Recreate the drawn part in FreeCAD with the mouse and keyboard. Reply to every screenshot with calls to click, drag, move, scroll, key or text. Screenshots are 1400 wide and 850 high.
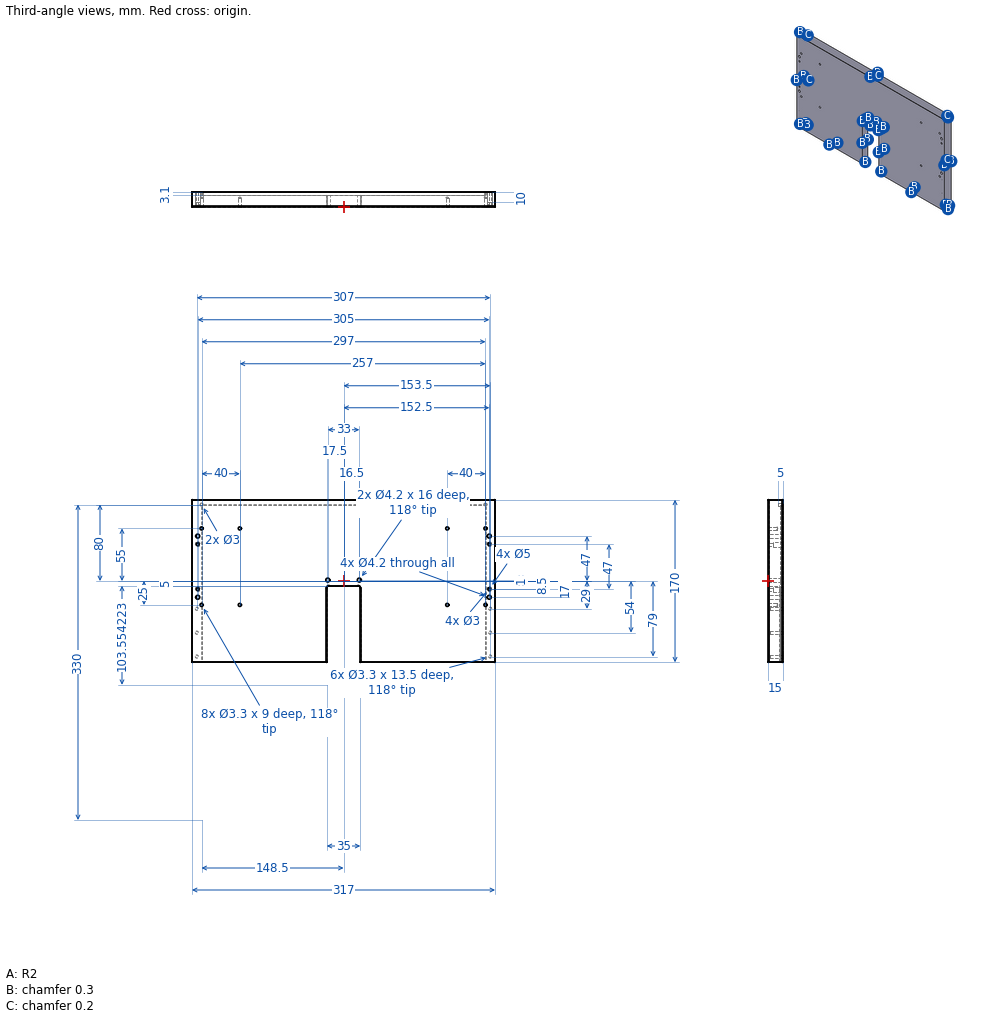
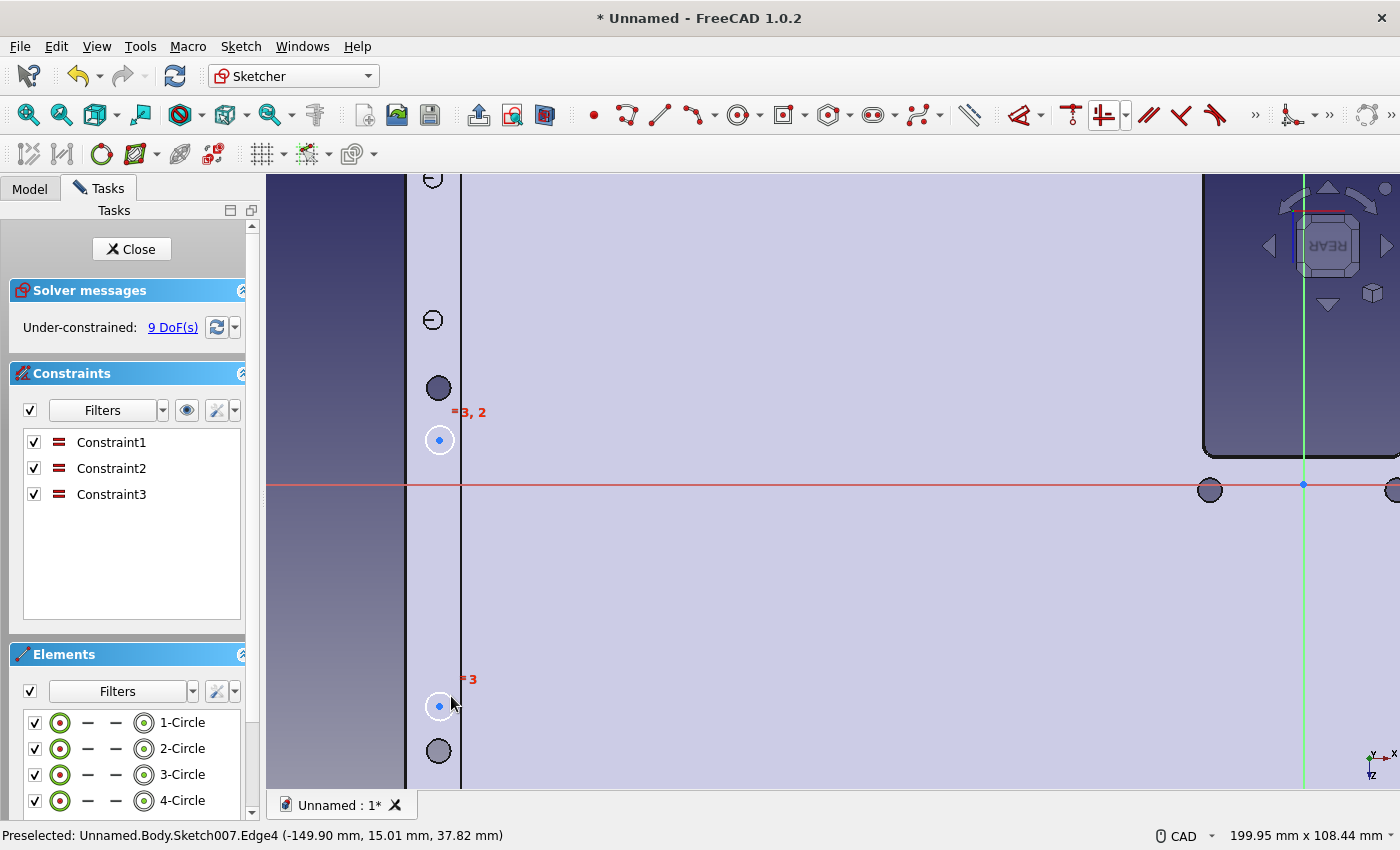
scroll(451, 430, down, 5)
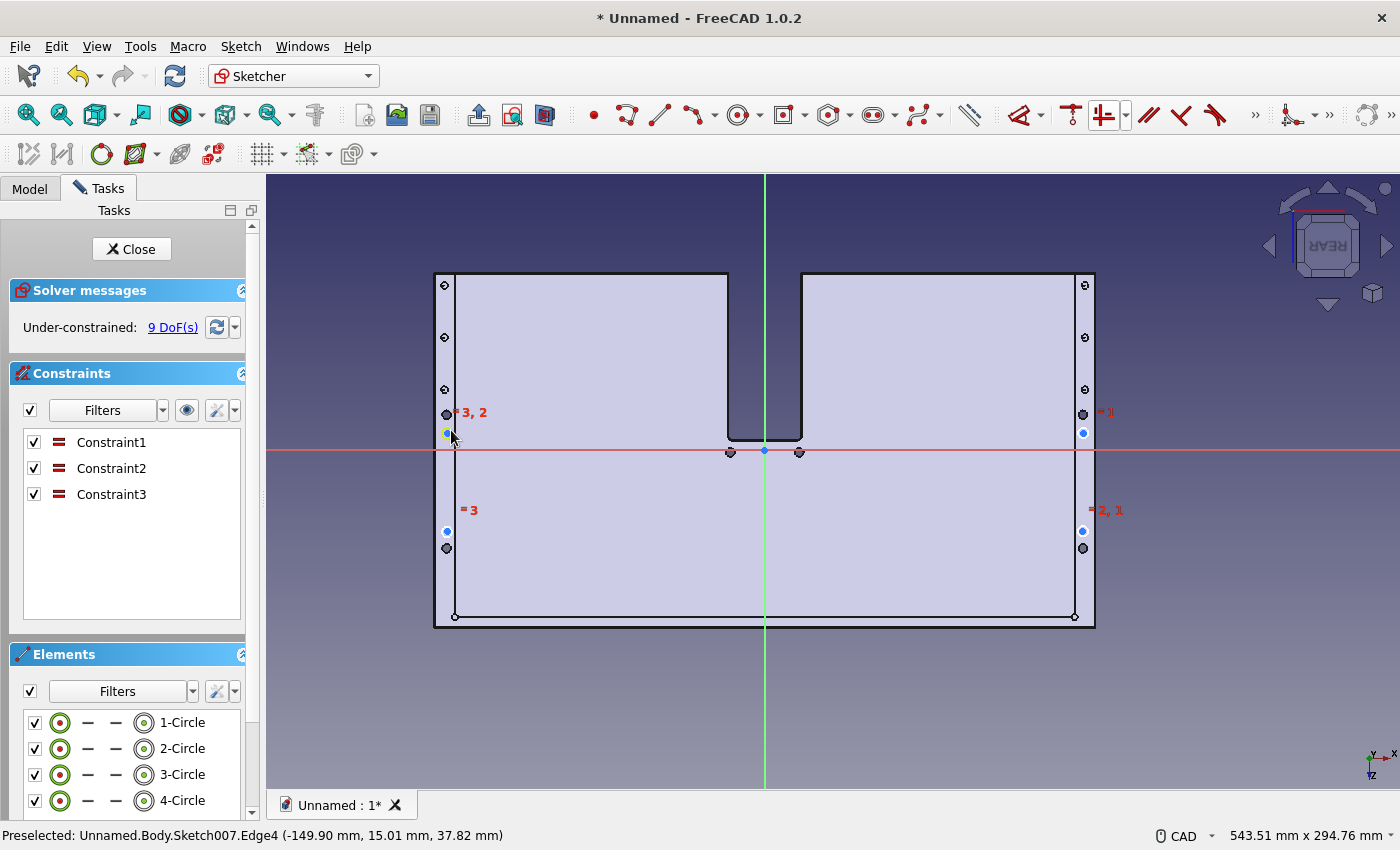
click(1083, 433)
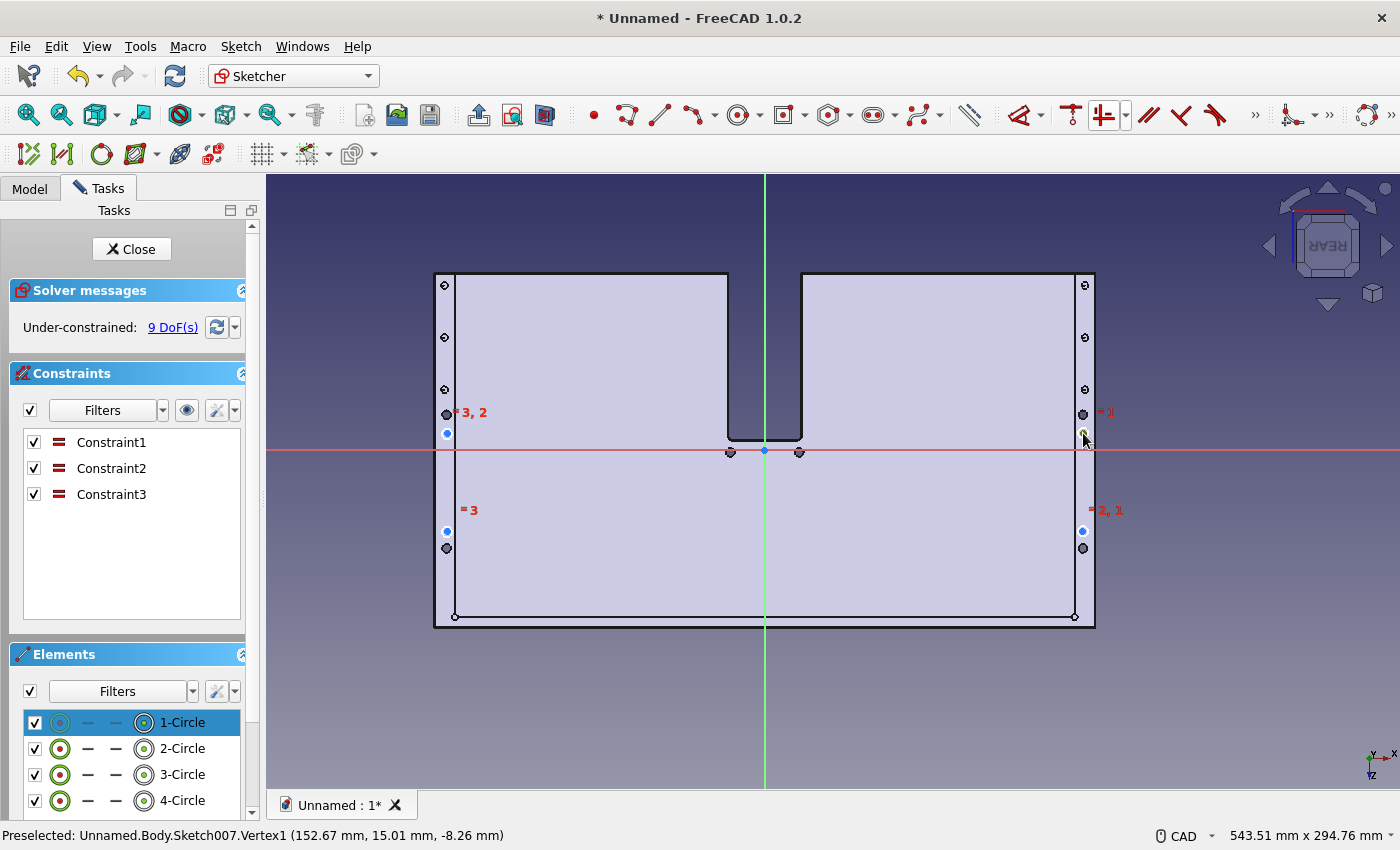
click(1083, 531)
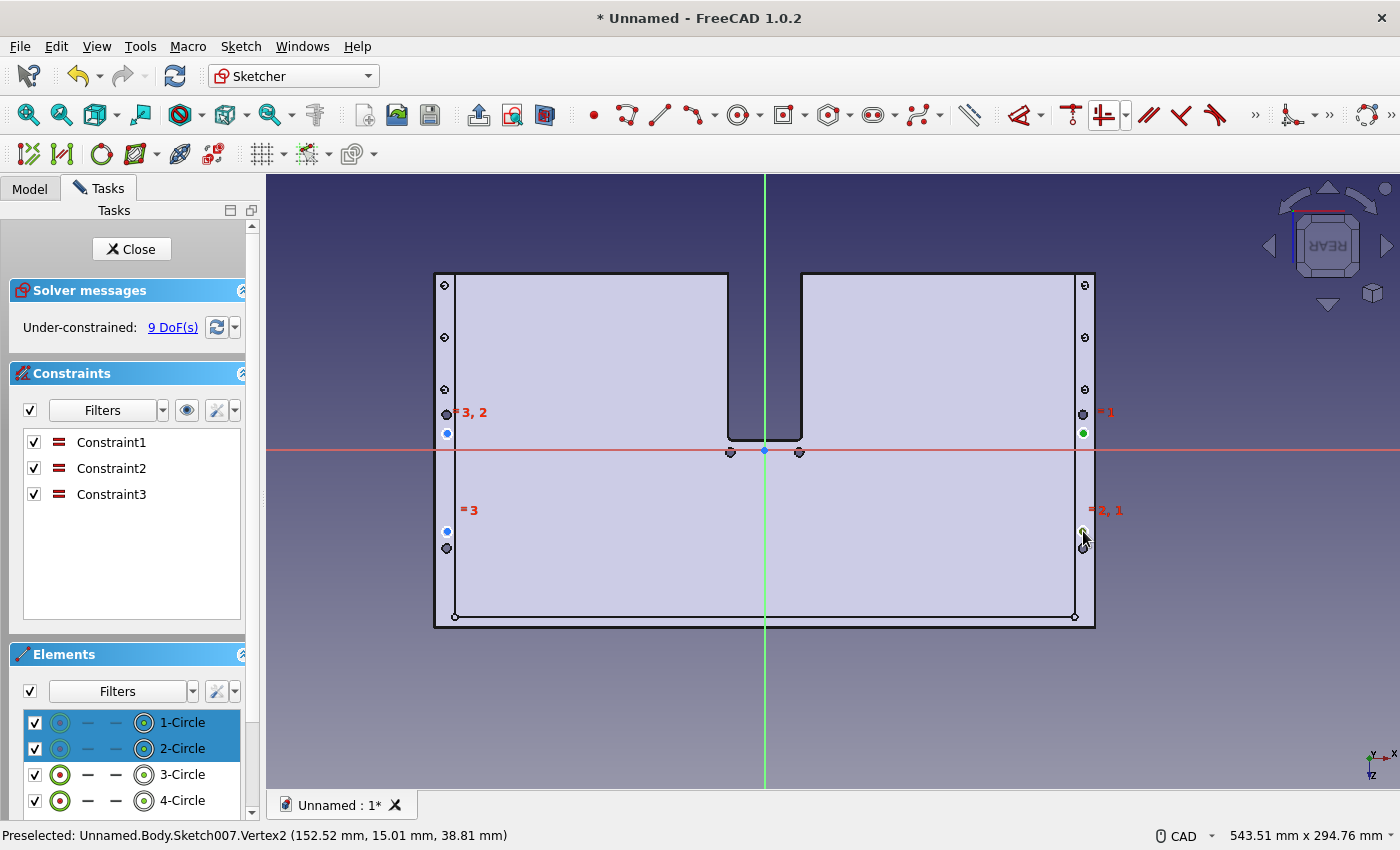
key(v)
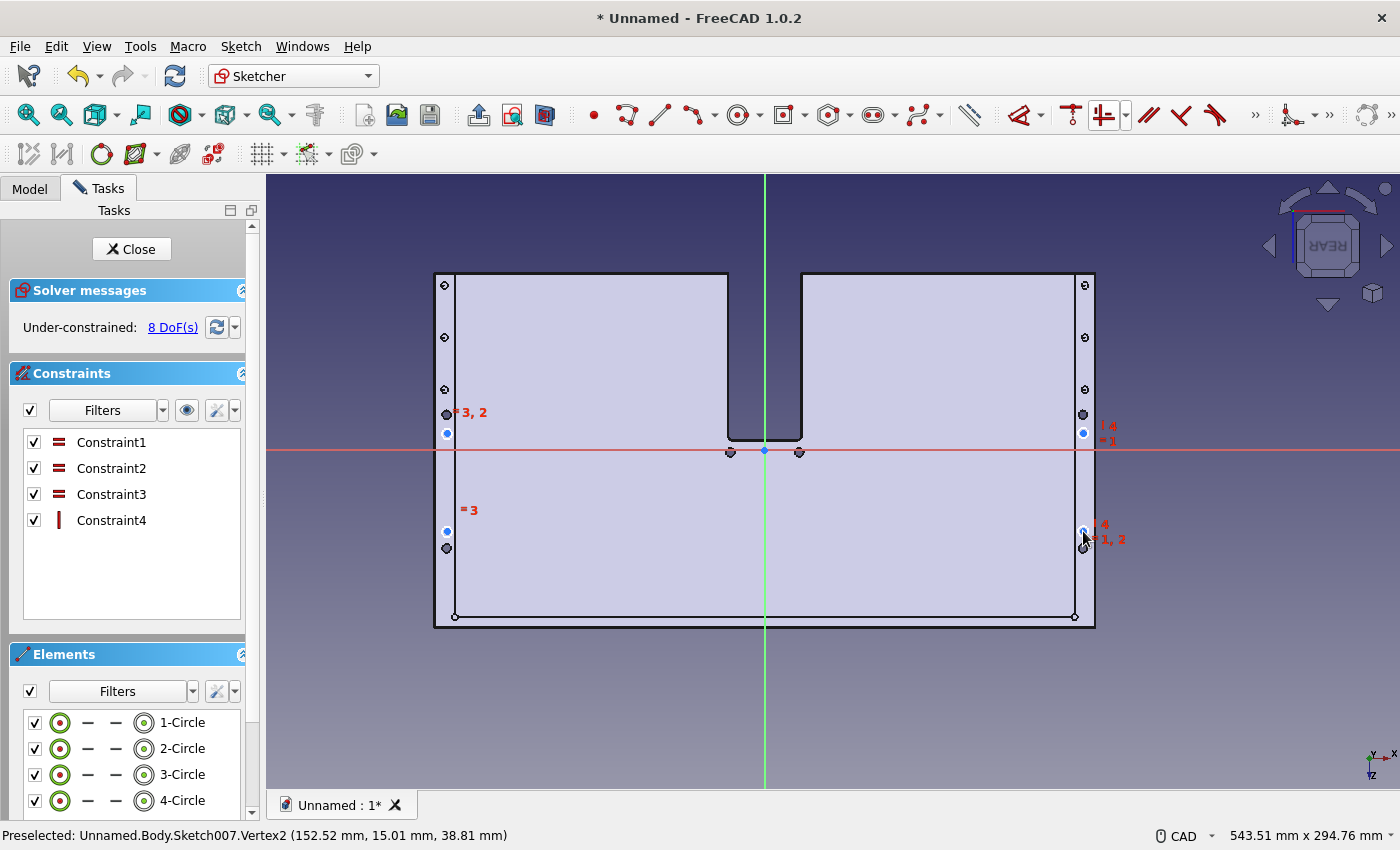
click(1083, 433)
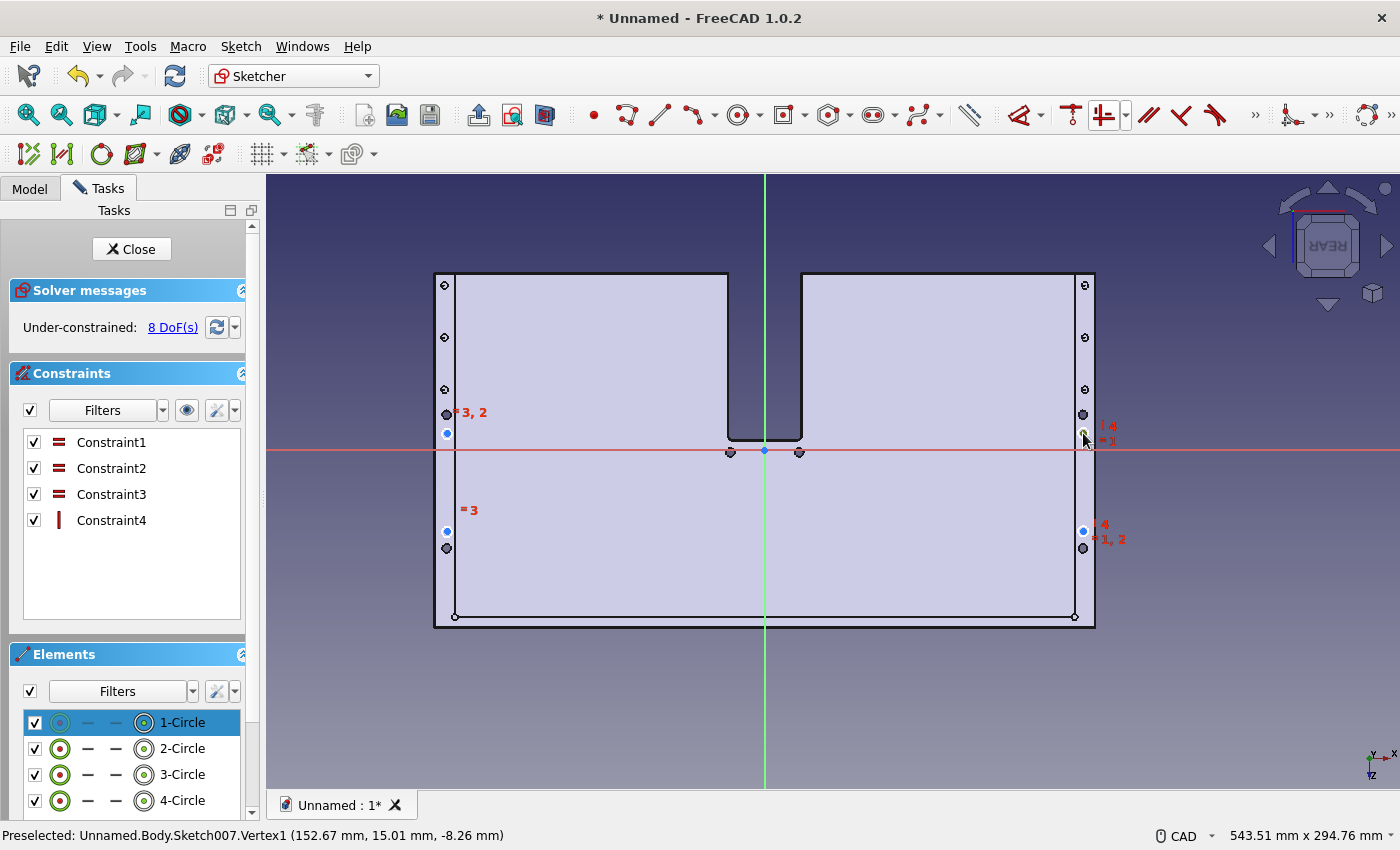
click(447, 434)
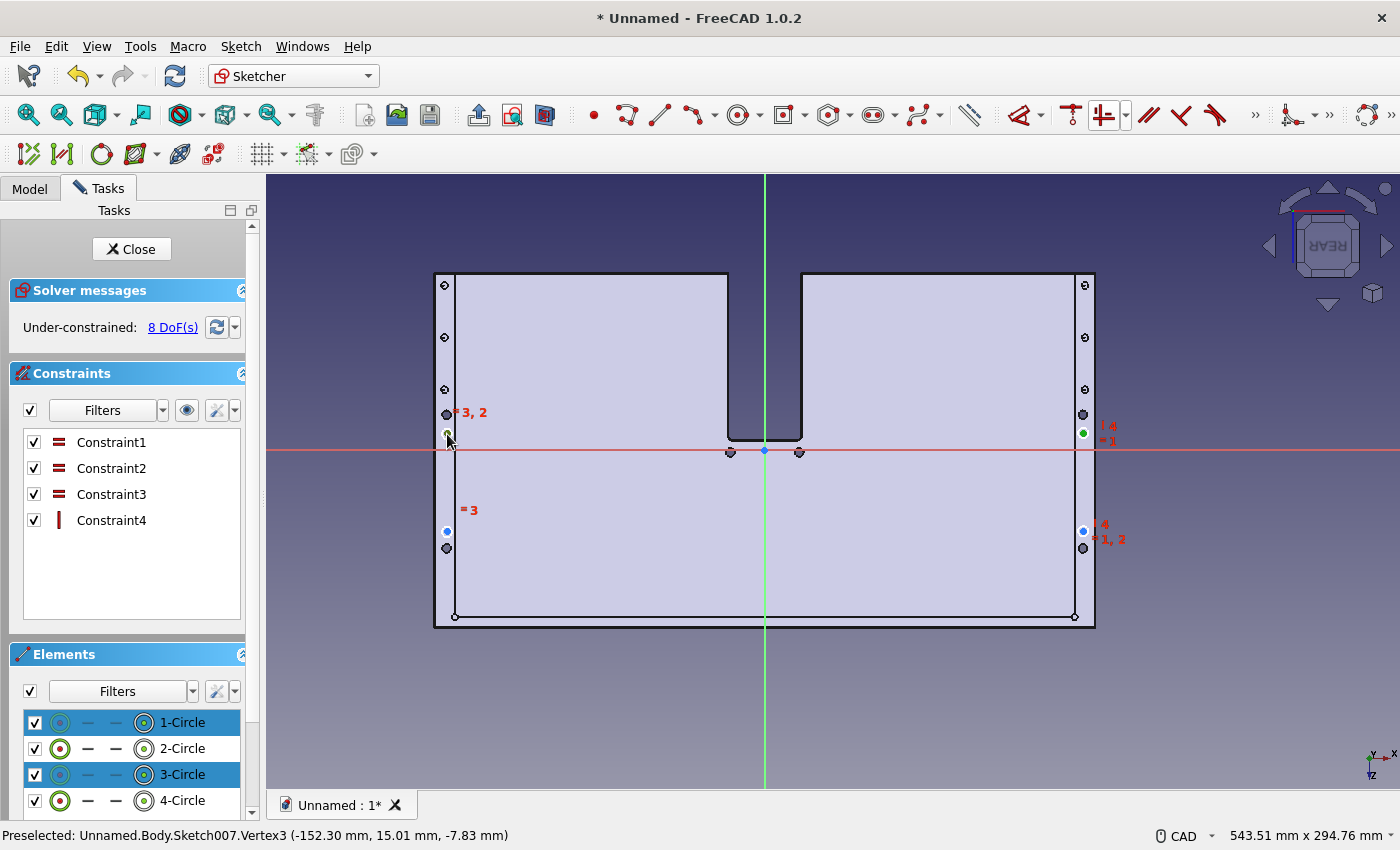
click(1126, 116)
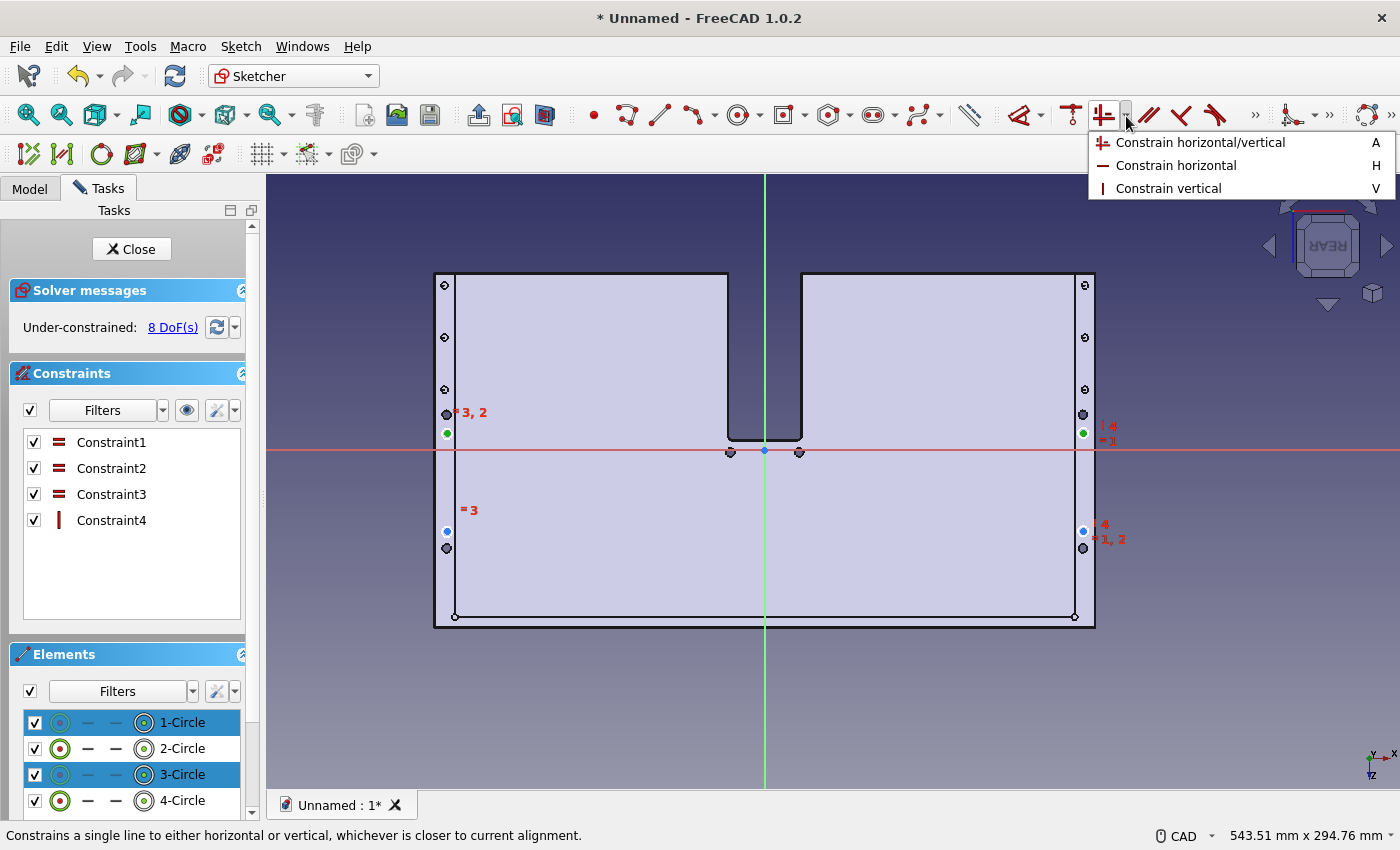
click(1242, 166)